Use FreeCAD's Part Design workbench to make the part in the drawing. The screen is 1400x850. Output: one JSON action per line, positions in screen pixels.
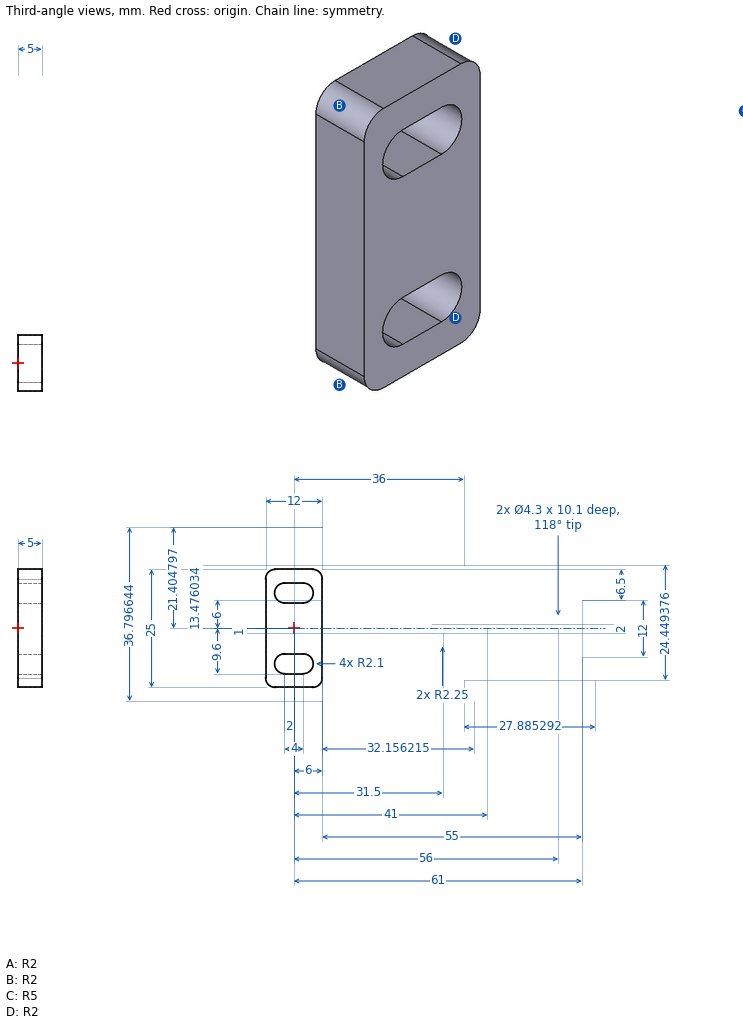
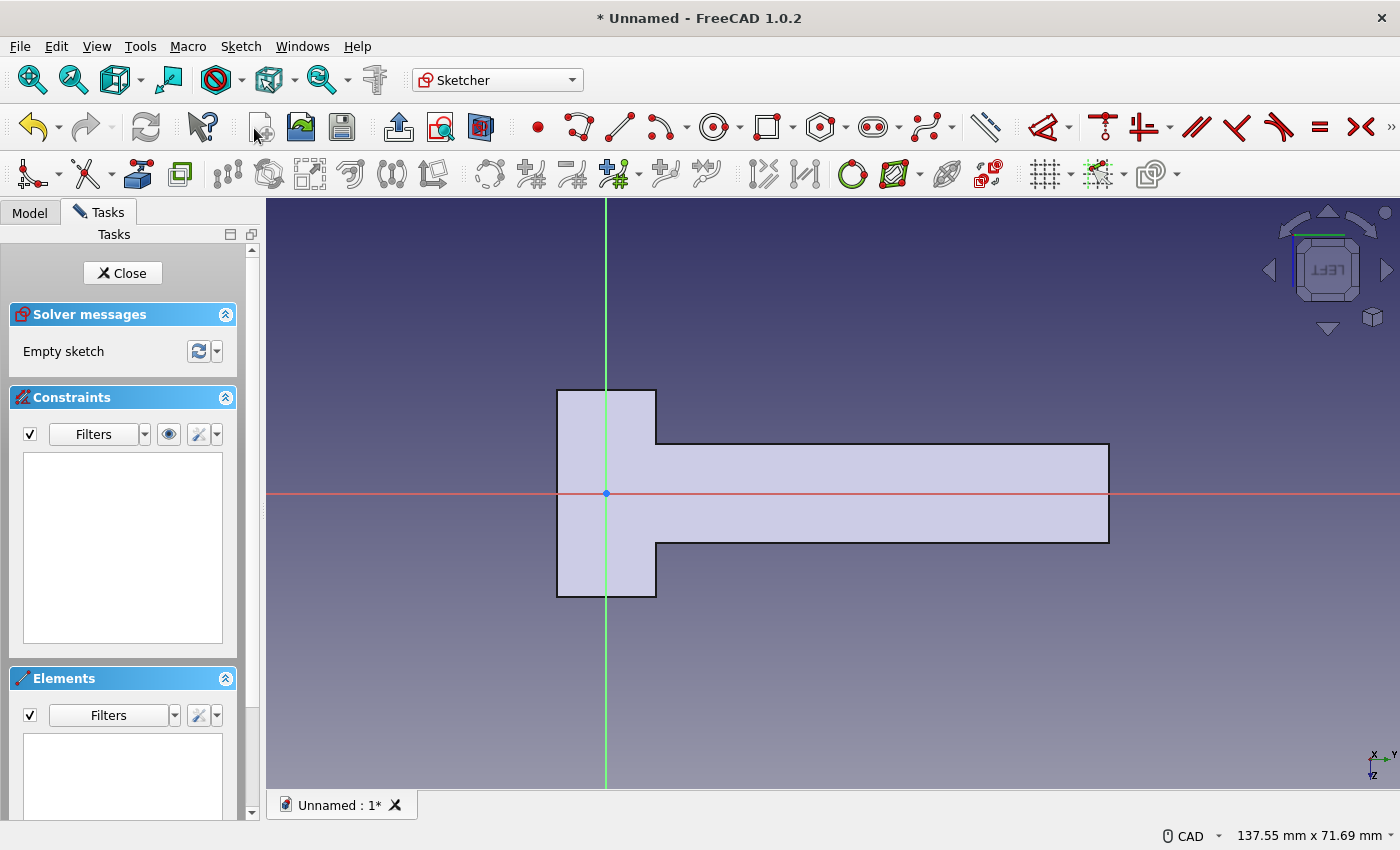
{"action": "left_click", "coordinate": [579, 128]}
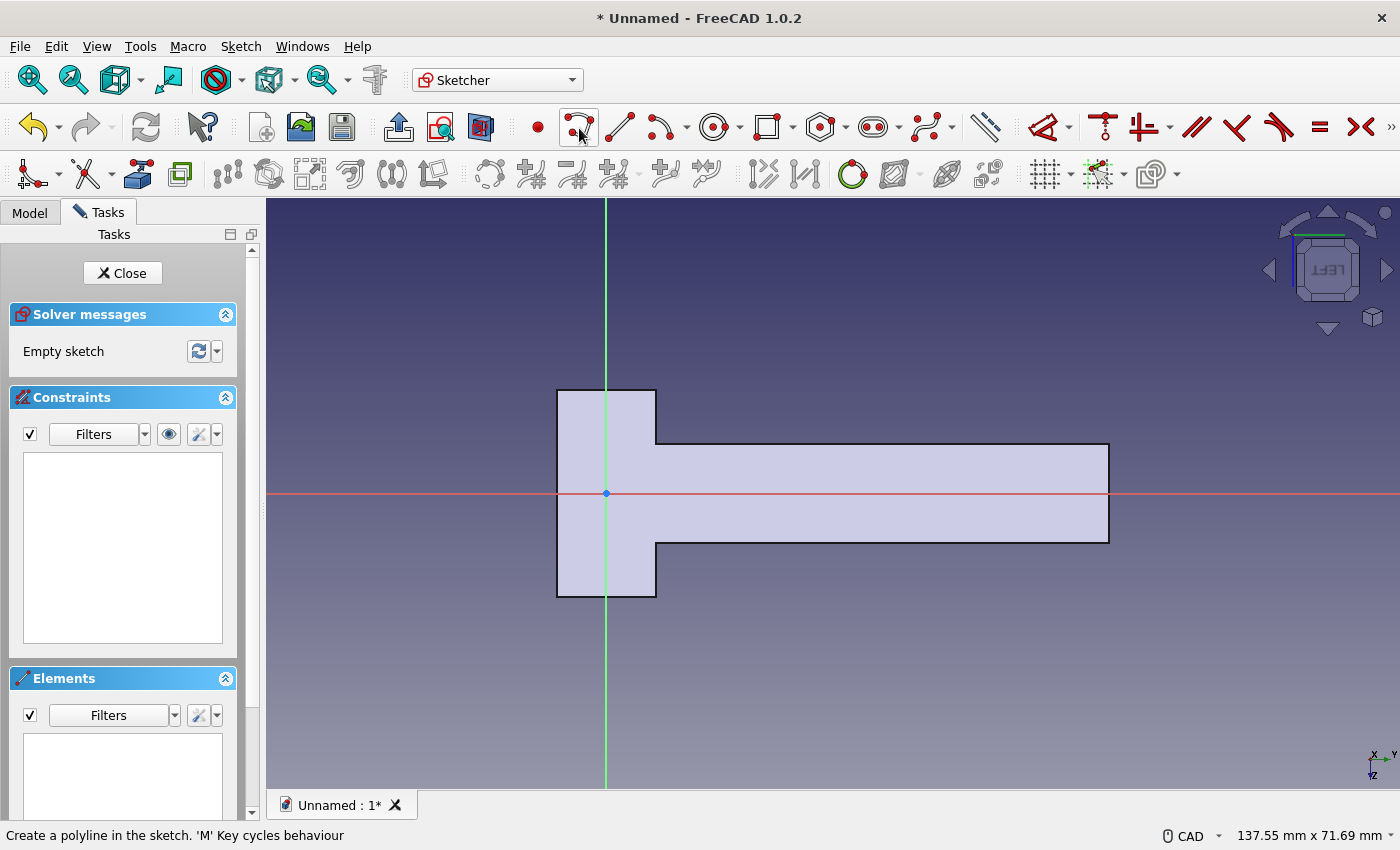
{"action": "left_click", "coordinate": [656, 390]}
{"action": "left_click", "coordinate": [656, 597]}
{"action": "left_click", "coordinate": [1109, 543]}
{"action": "left_click", "coordinate": [1109, 444]}
{"action": "left_click", "coordinate": [656, 391]}
{"action": "key", "text": "Escape"}
{"action": "key", "text": "Escape"}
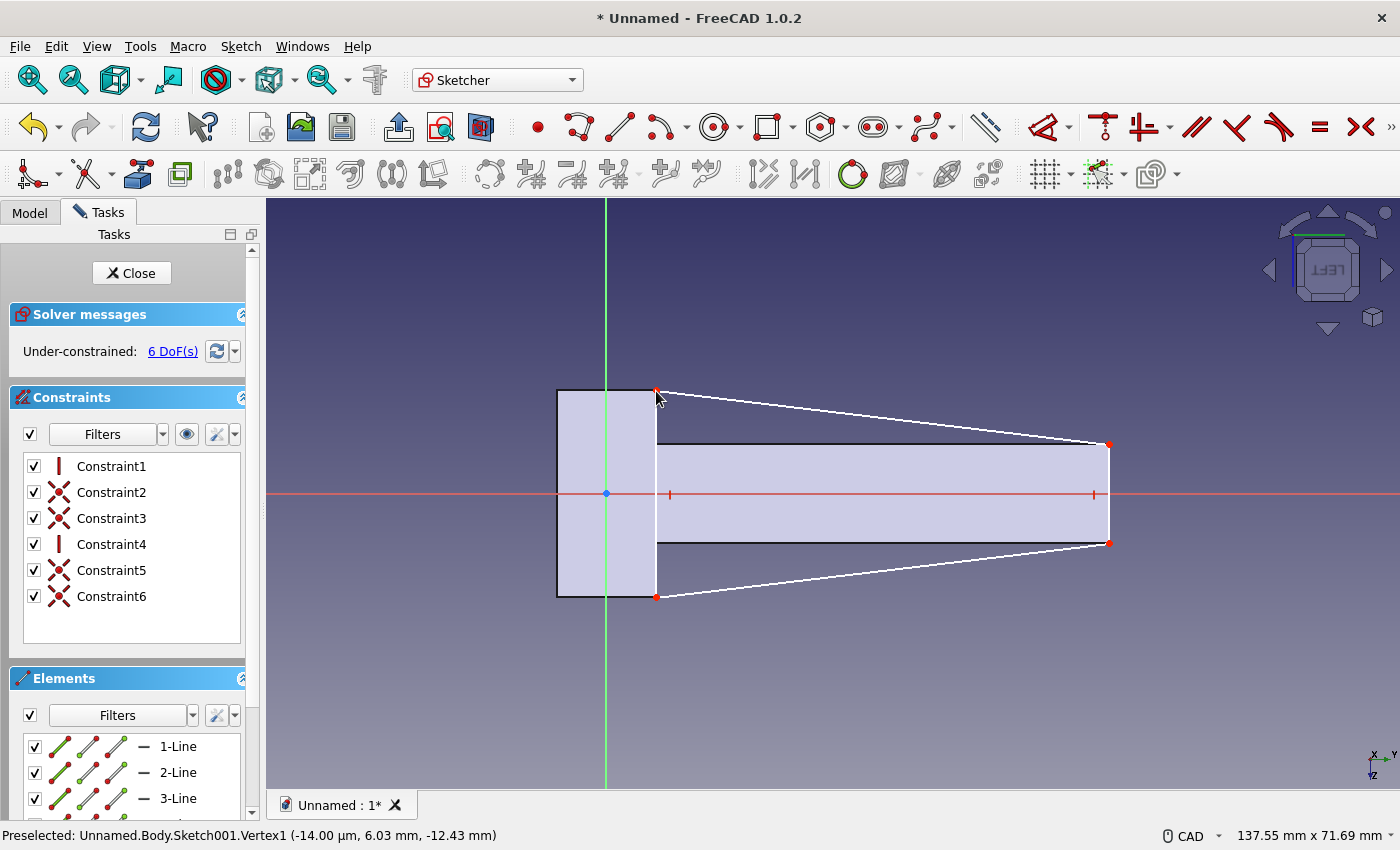
{"action": "left_click", "coordinate": [1042, 128]}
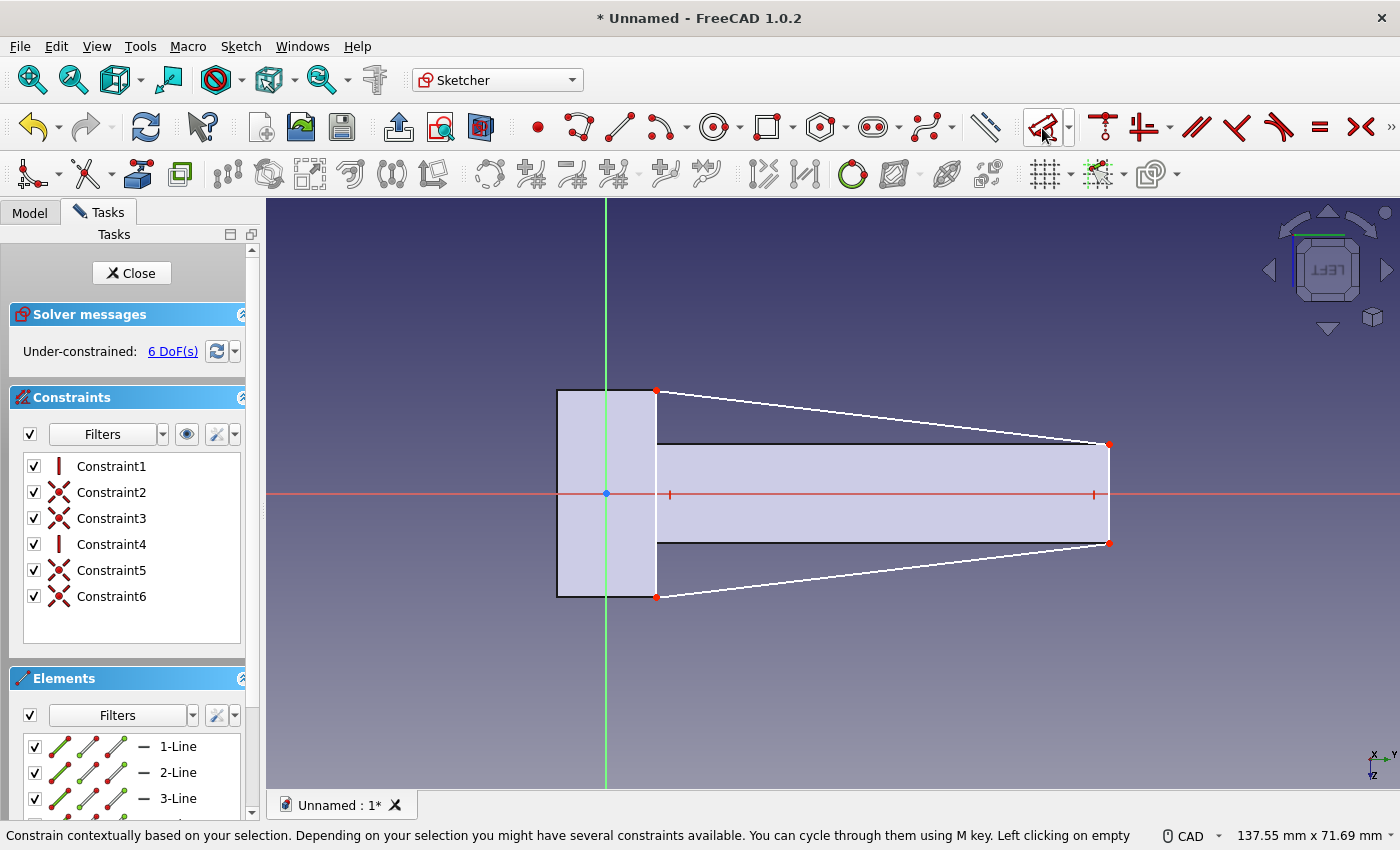
{"action": "left_click", "coordinate": [656, 453]}
{"action": "left_click", "coordinate": [622, 447]}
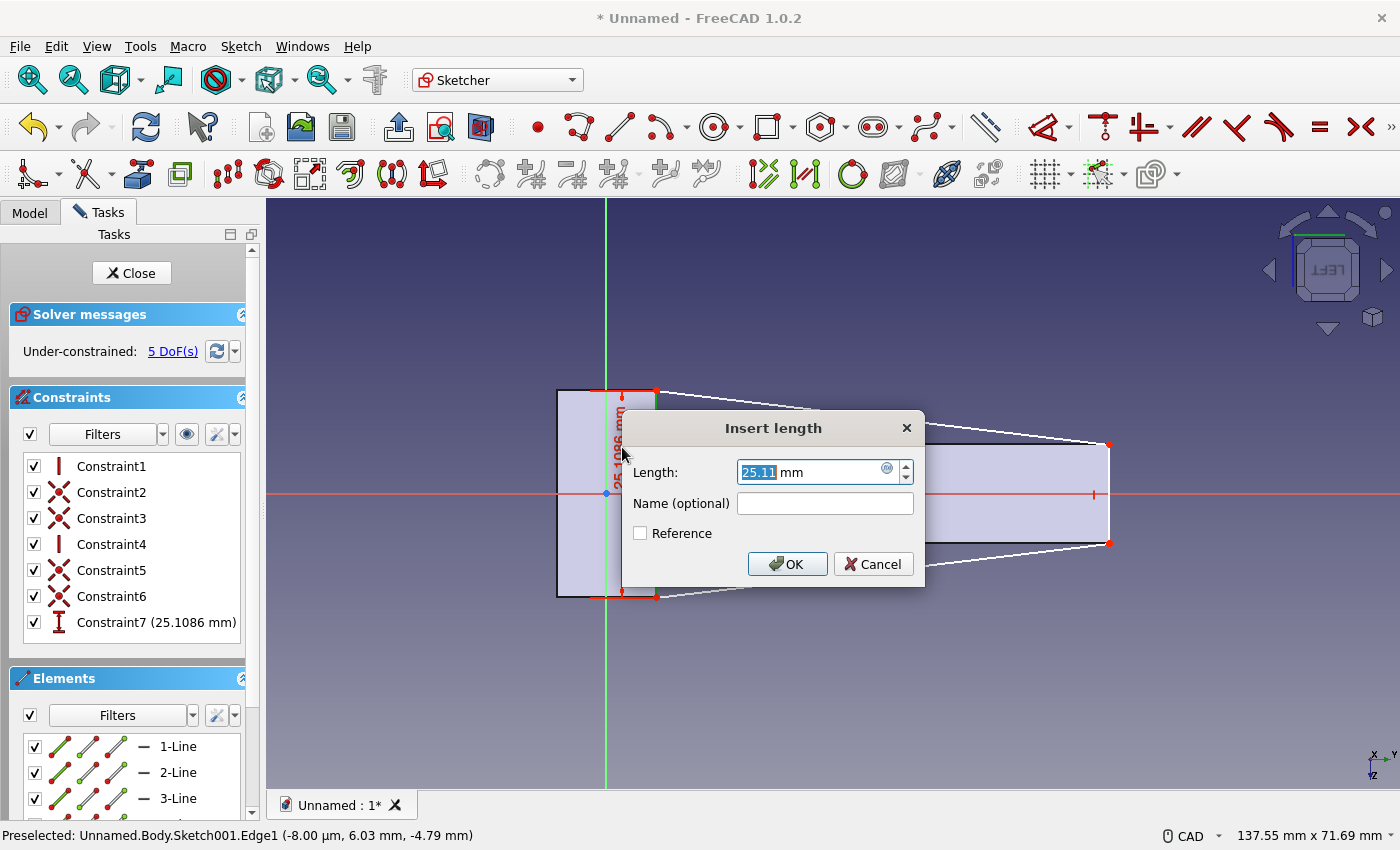
{"action": "type", "text": "25"}
{"action": "key", "text": "Return"}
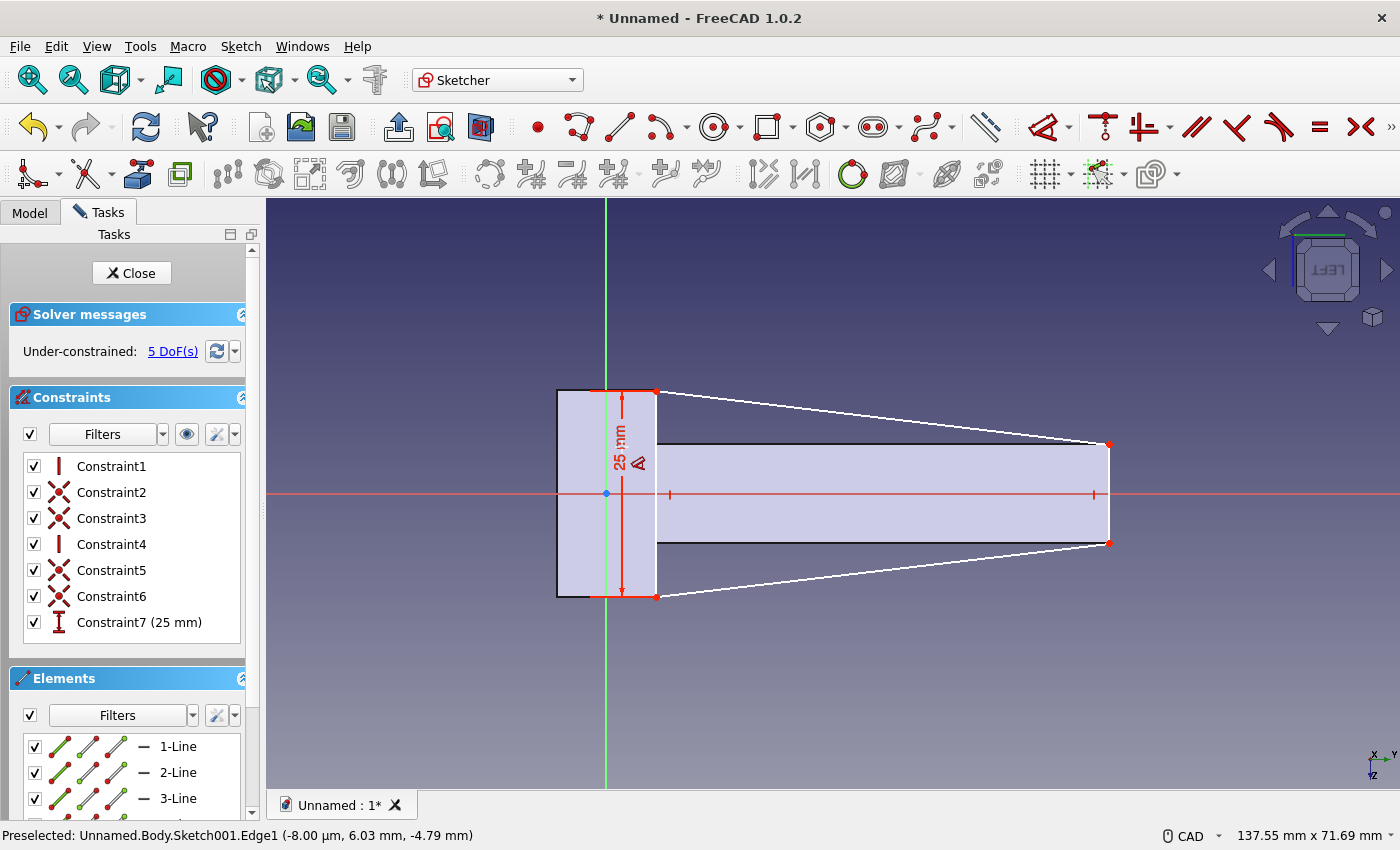
{"action": "left_click", "coordinate": [1109, 514]}
{"action": "left_click", "coordinate": [1143, 472]}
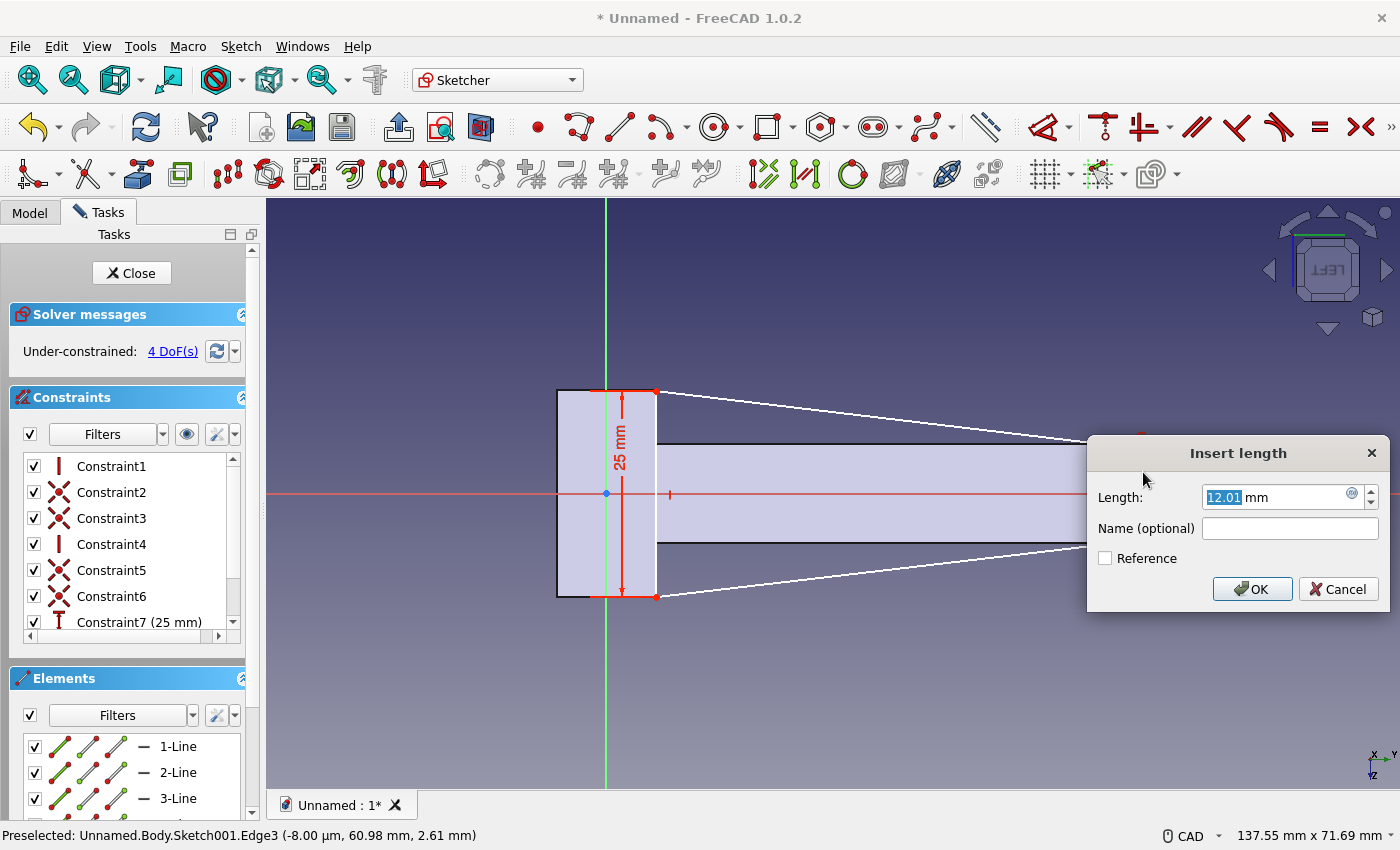
{"action": "type", "text": "12"}
{"action": "key", "text": "Return"}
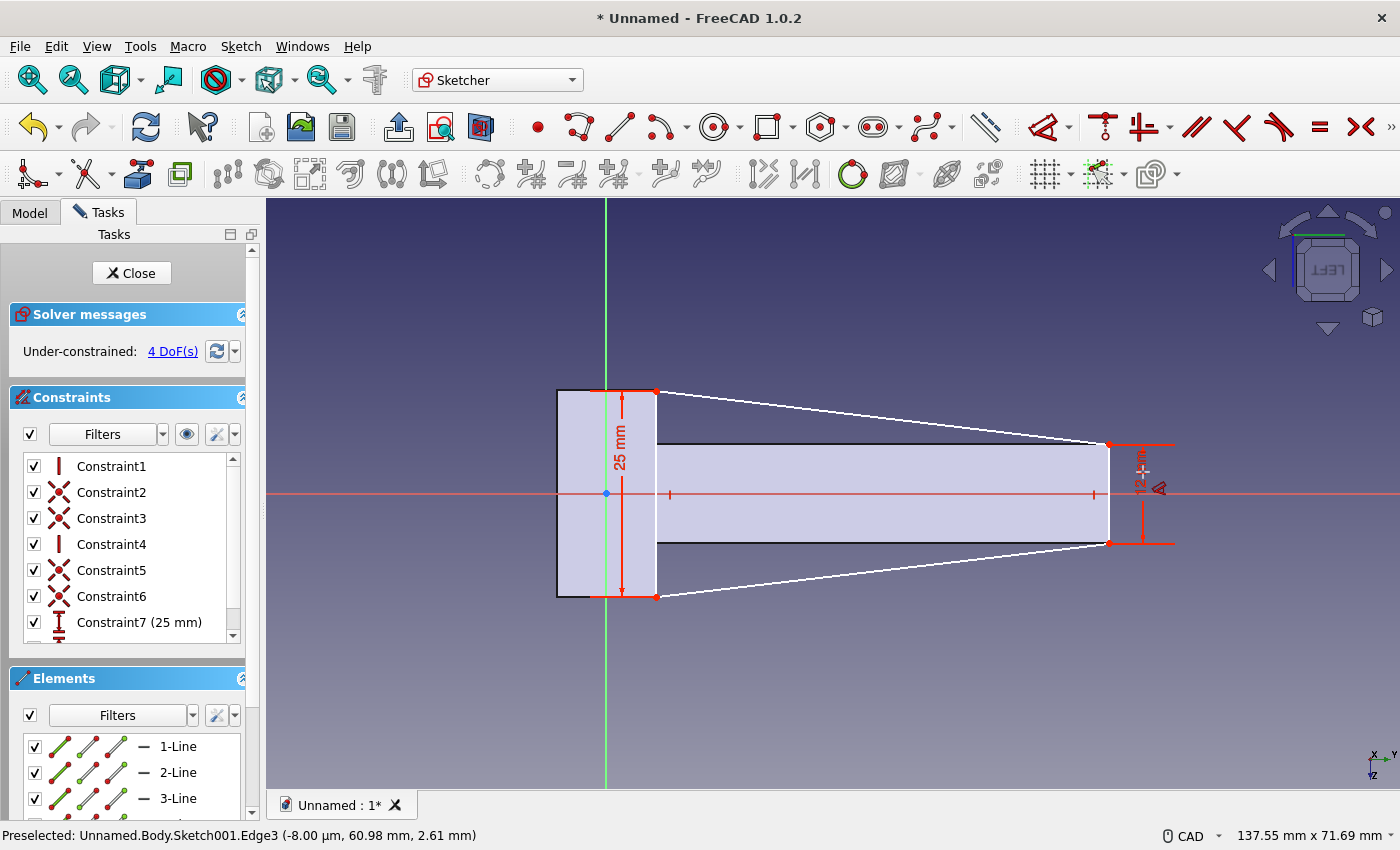
{"action": "left_click", "coordinate": [656, 391]}
{"action": "left_click", "coordinate": [631, 357]}